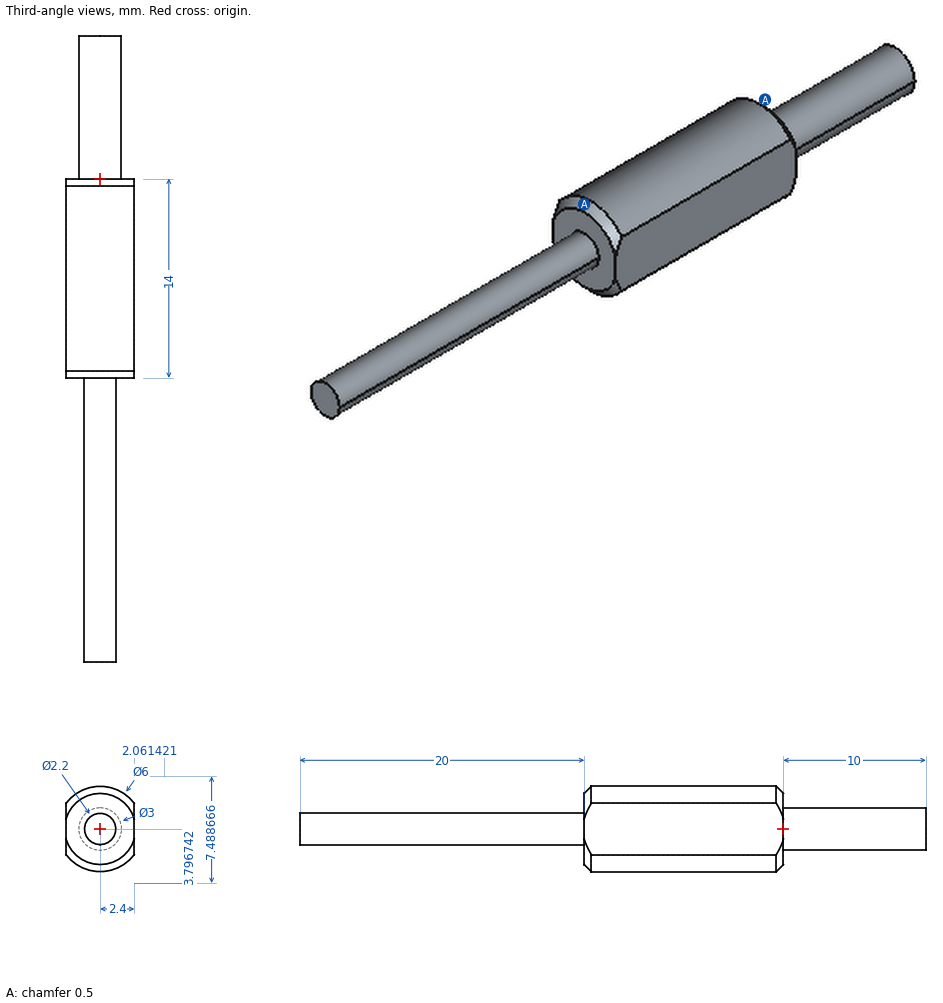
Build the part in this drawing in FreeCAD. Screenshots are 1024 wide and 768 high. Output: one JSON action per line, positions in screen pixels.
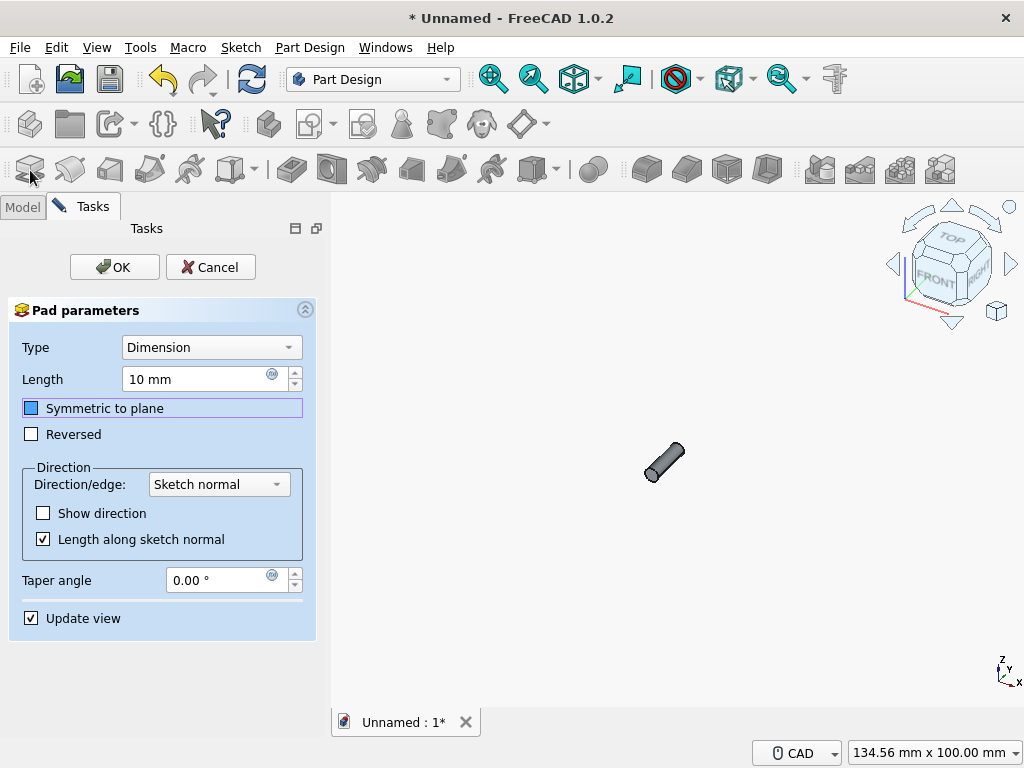
{"action": "left_click", "coordinate": [30, 434]}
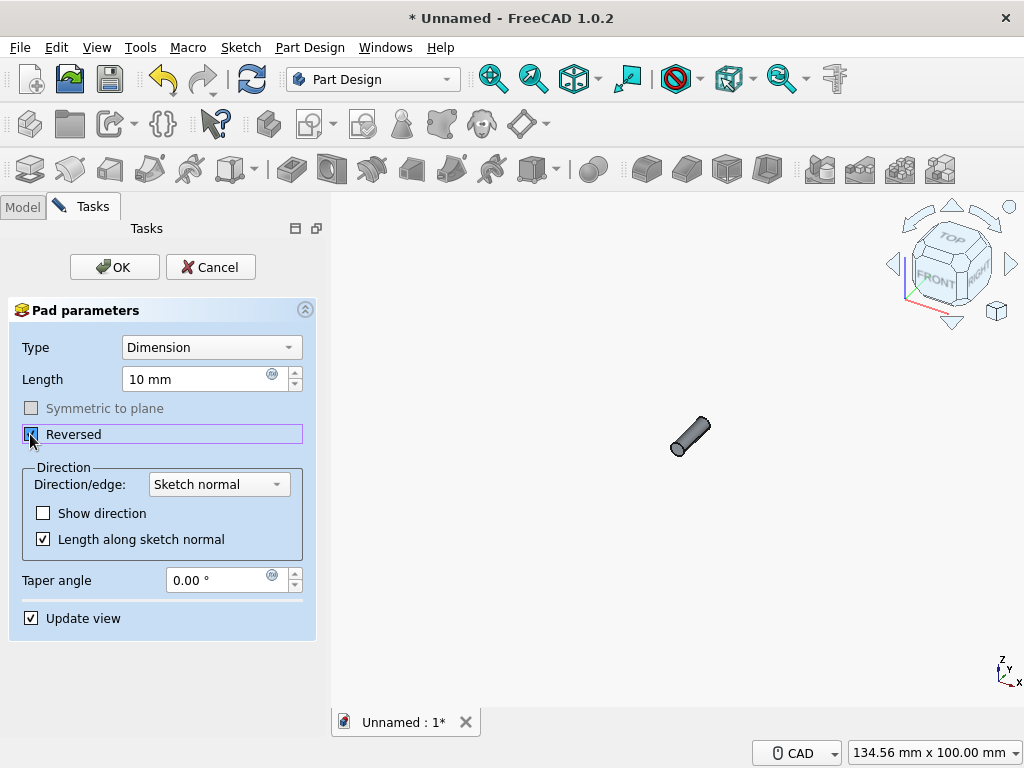
{"action": "left_click", "coordinate": [115, 267]}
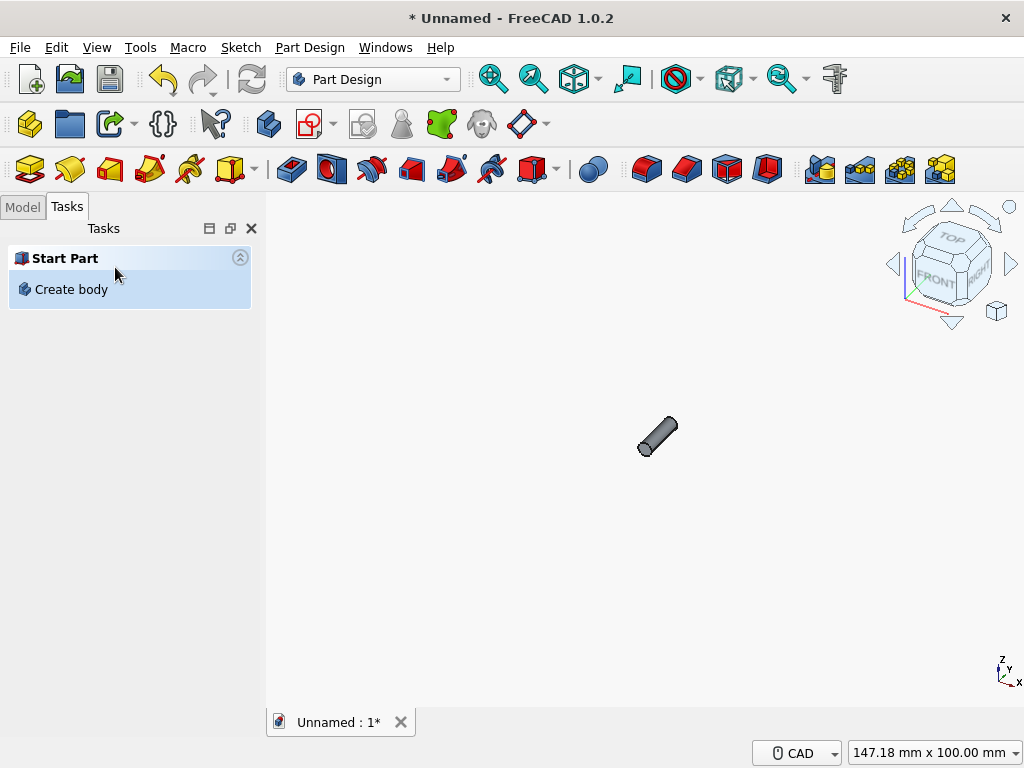
{"action": "key", "text": "v f"}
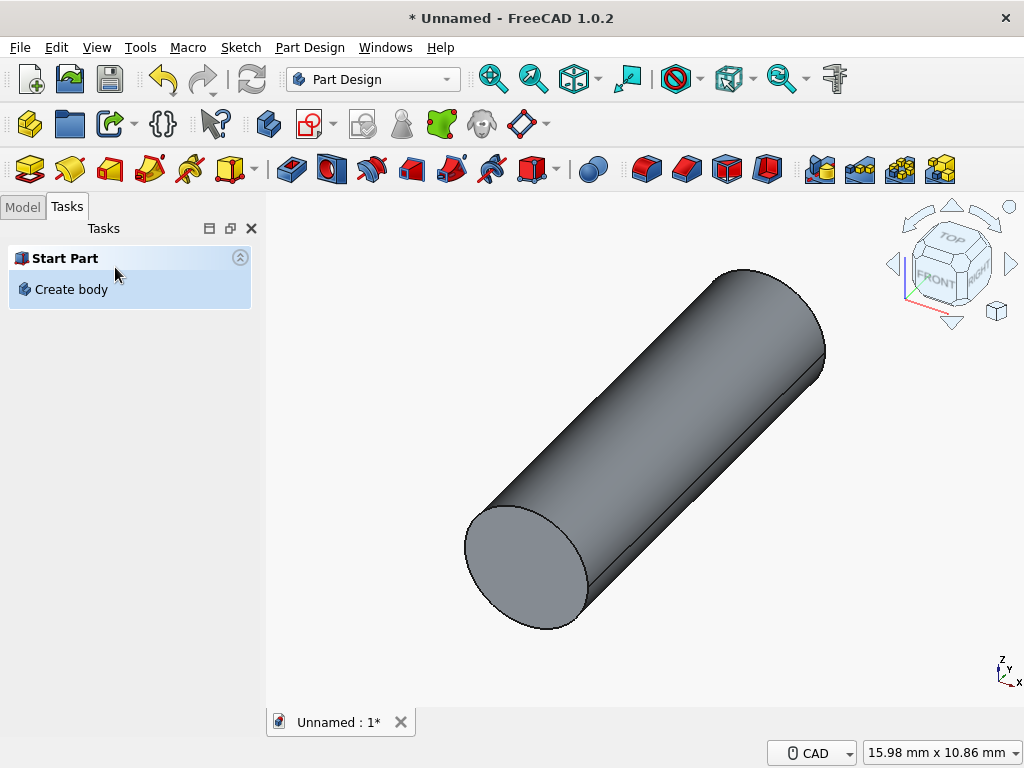
{"action": "left_click", "coordinate": [310, 124]}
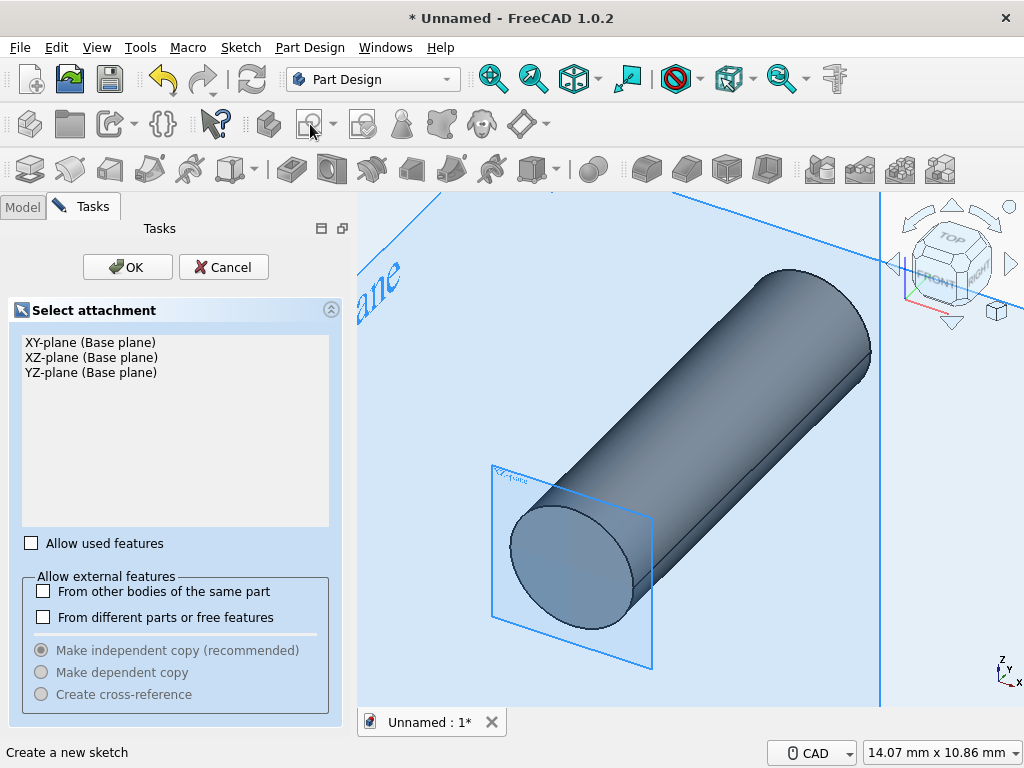
{"action": "left_click", "coordinate": [82, 358]}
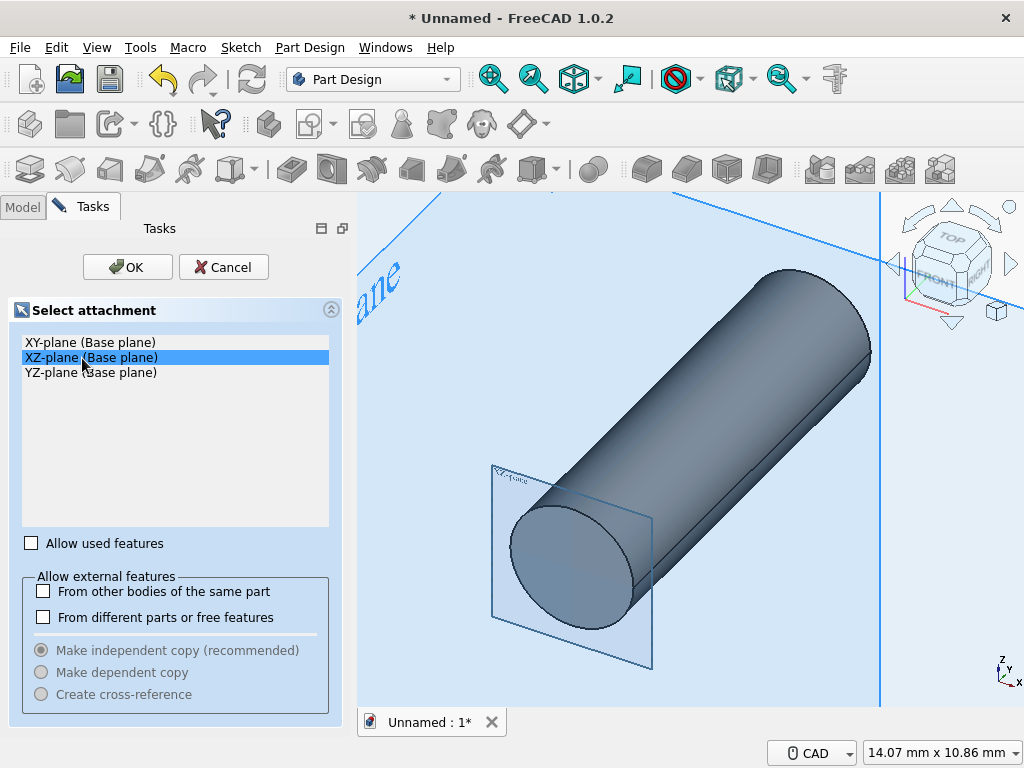
{"action": "left_click", "coordinate": [128, 267]}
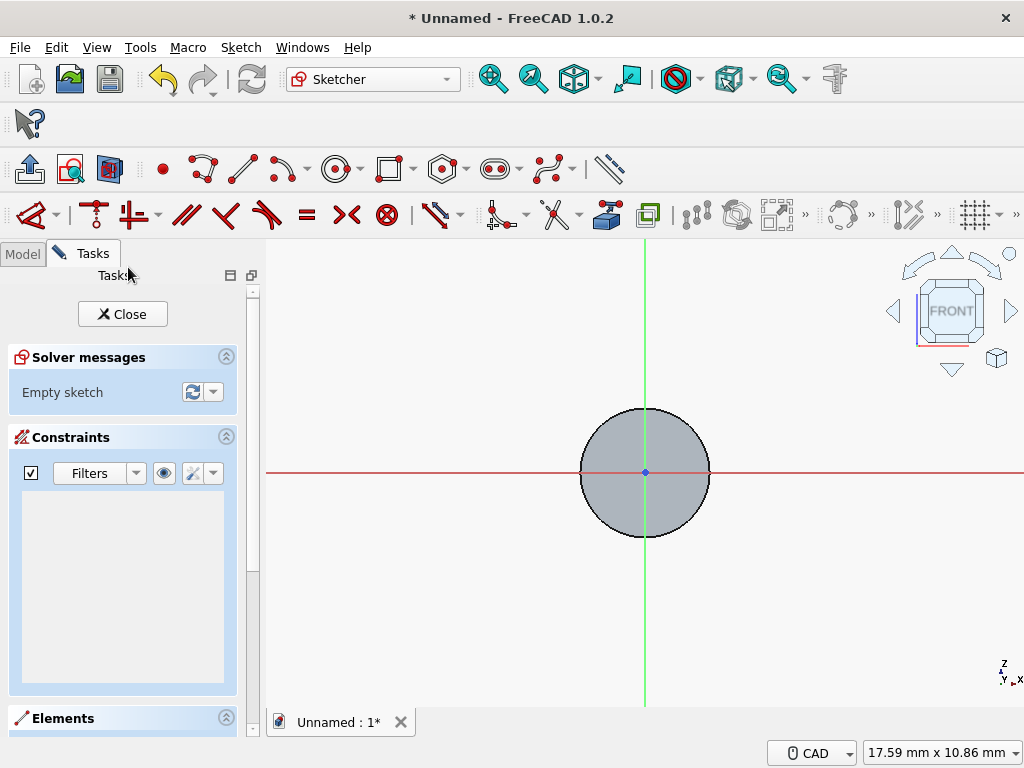
{"action": "left_click", "coordinate": [336, 170]}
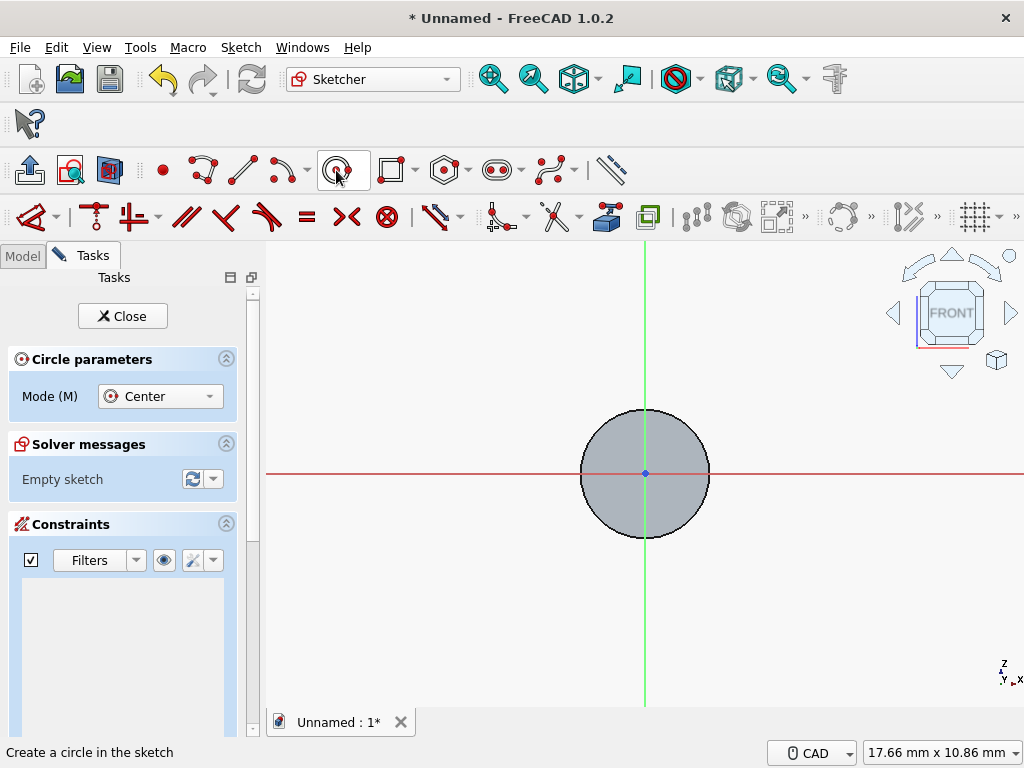
{"action": "left_click", "coordinate": [645, 474]}
{"action": "left_click", "coordinate": [736, 383]}
{"action": "key", "text": "Escape"}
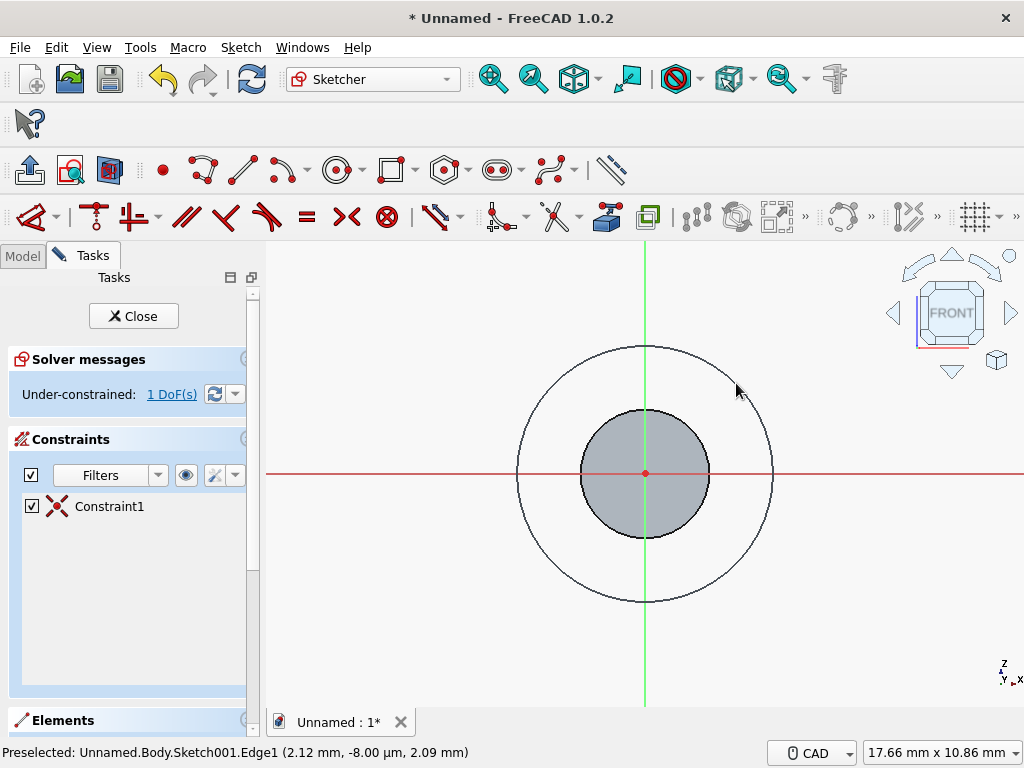
{"action": "left_click", "coordinate": [32, 218]}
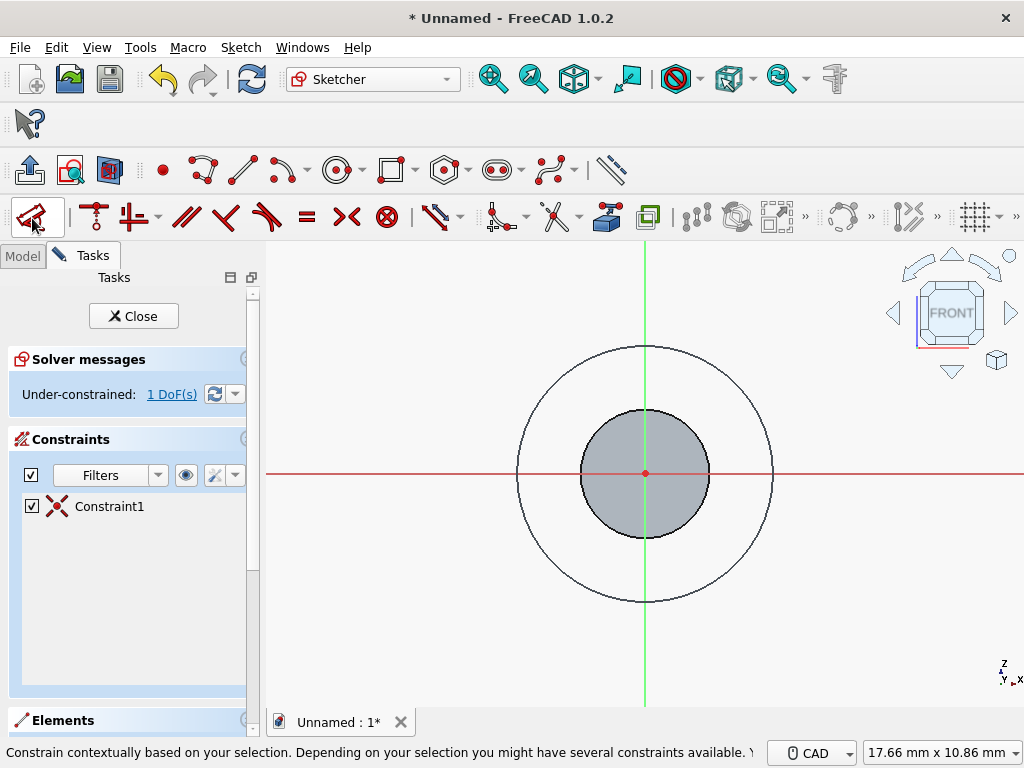
{"action": "left_click", "coordinate": [735, 383]}
{"action": "left_click", "coordinate": [758, 360]}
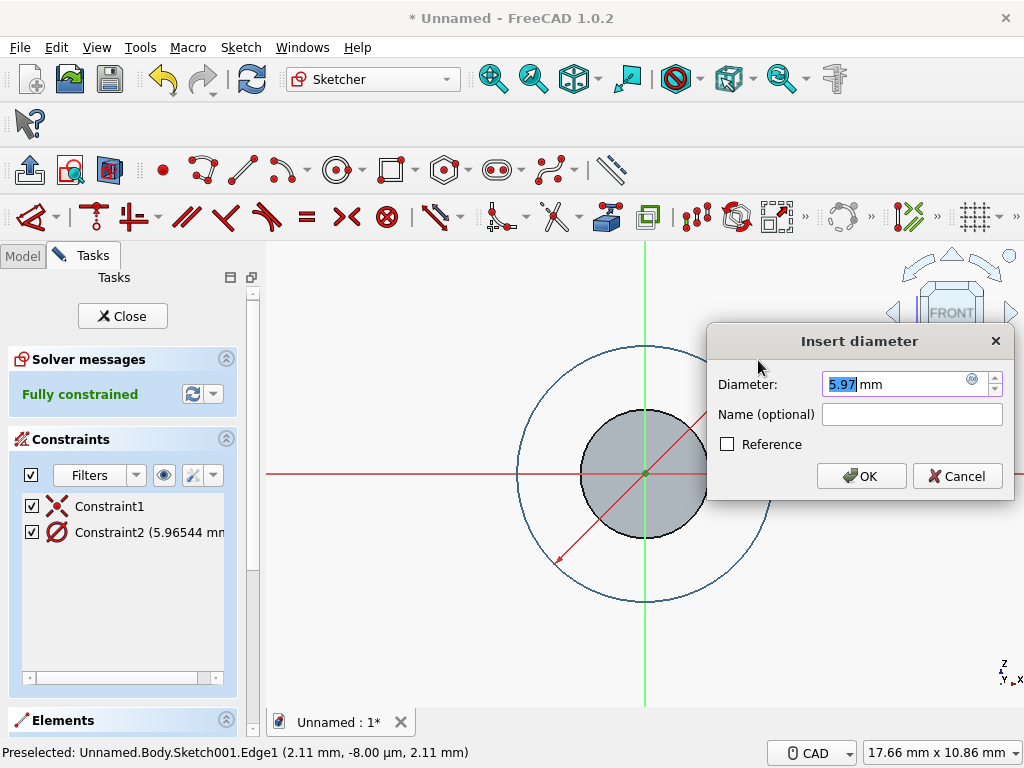
{"action": "type", "text": "6"}
{"action": "key", "text": "Return"}
{"action": "key", "text": "Escape"}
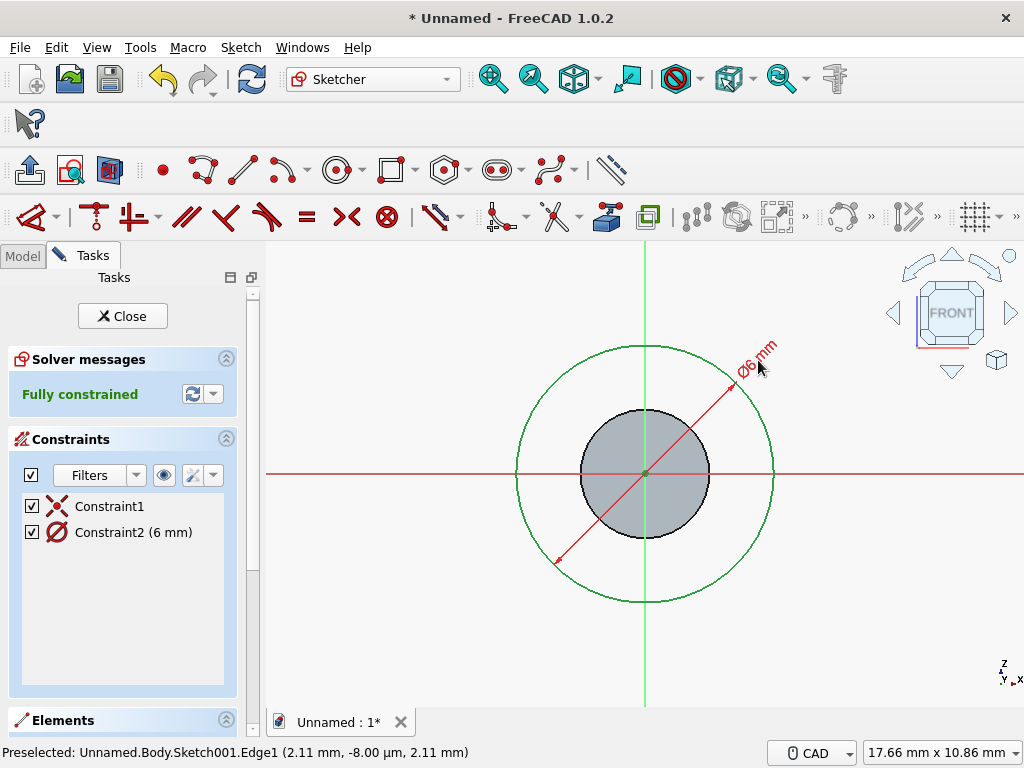
{"action": "left_click", "coordinate": [123, 316]}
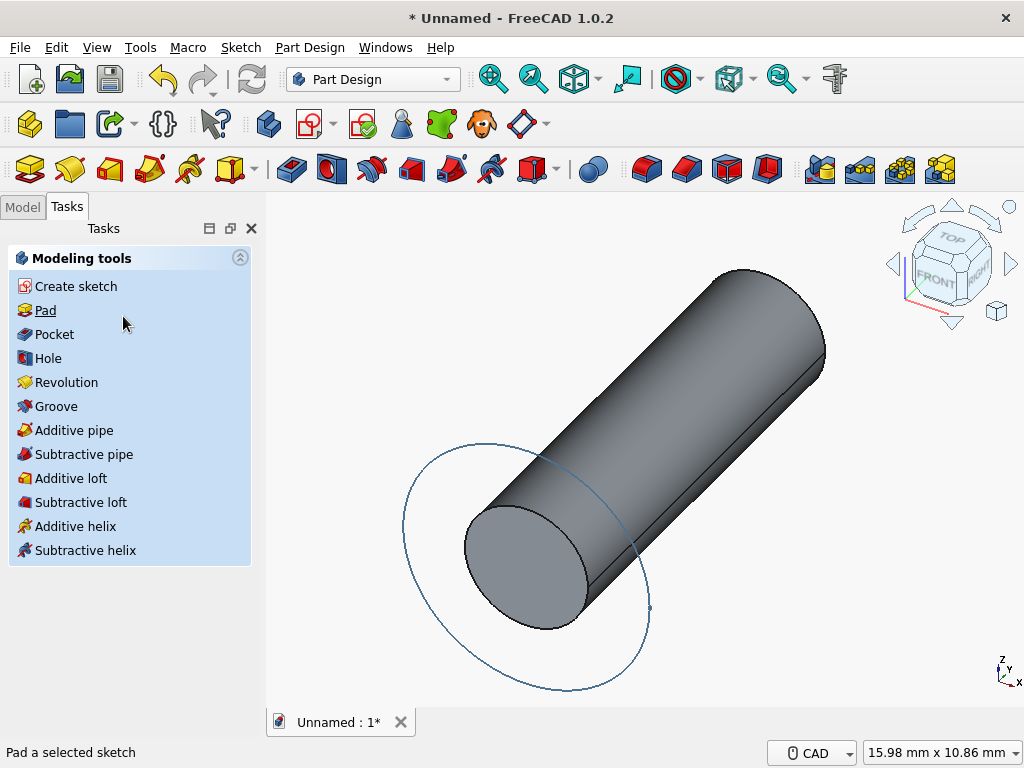
{"action": "left_click", "coordinate": [30, 170]}